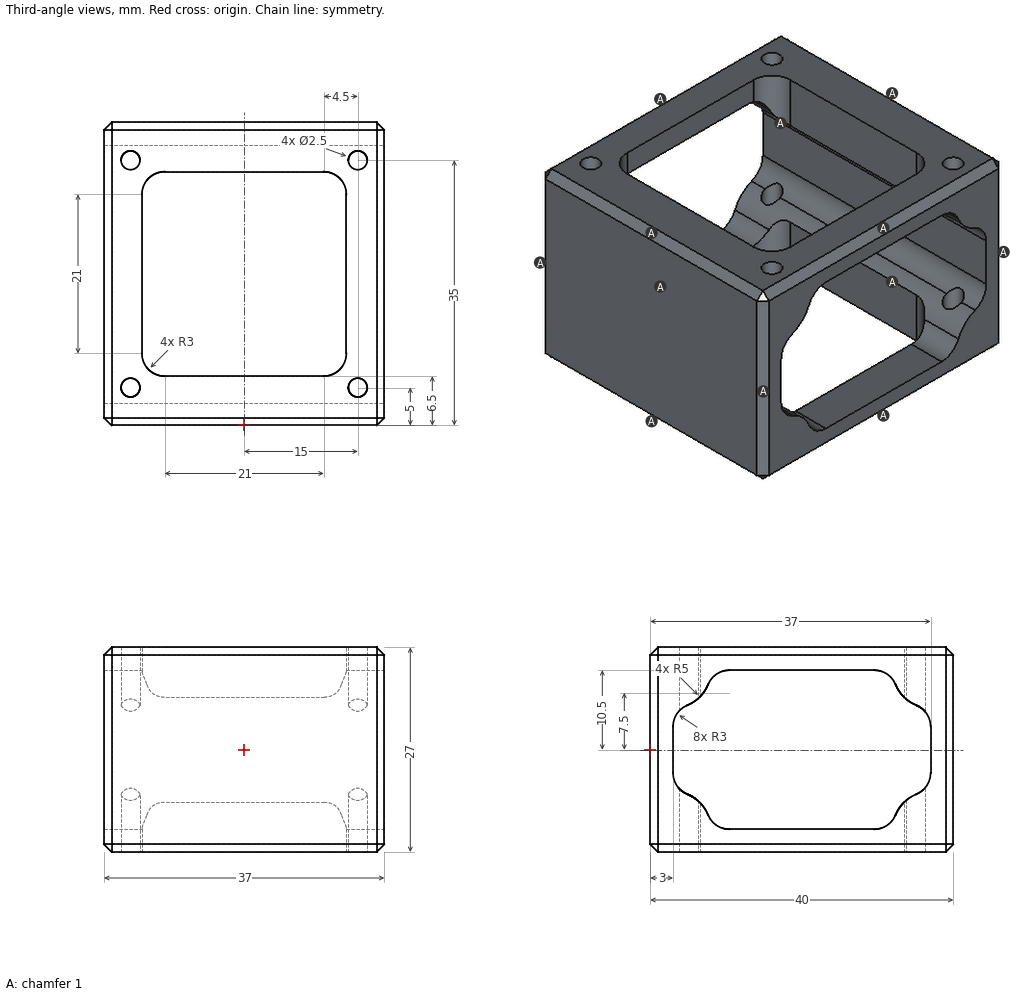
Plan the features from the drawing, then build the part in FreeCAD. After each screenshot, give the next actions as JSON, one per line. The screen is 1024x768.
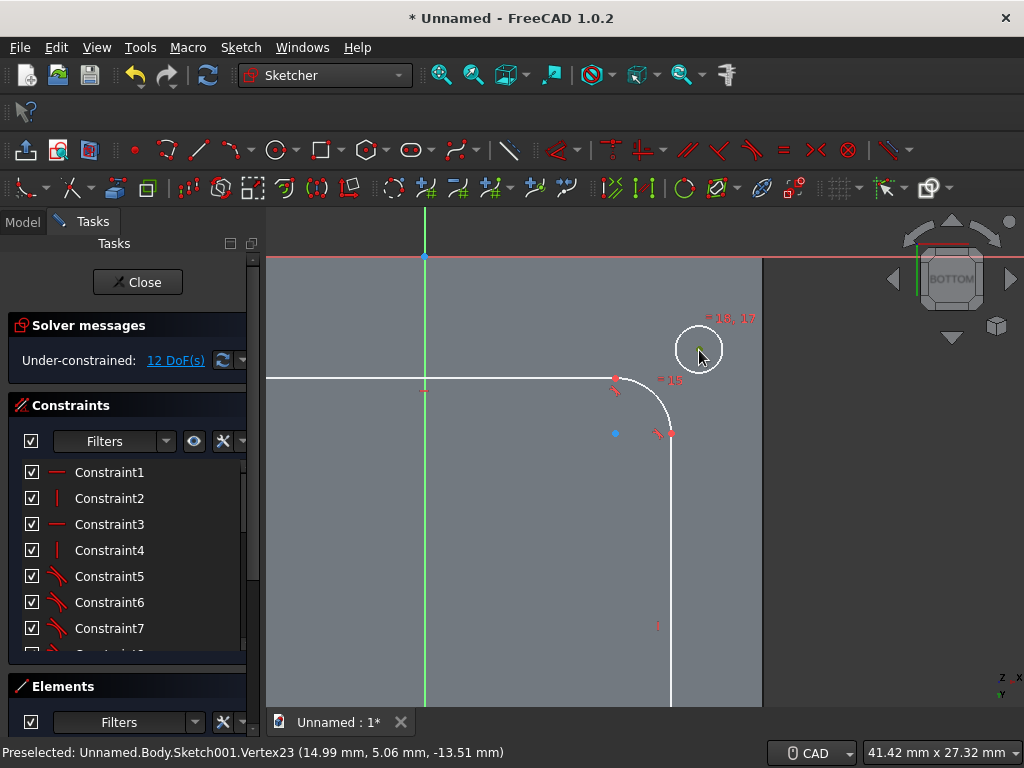
{"action": "scroll", "coordinate": [700, 350], "scroll_direction": "down", "scroll_amount": 4}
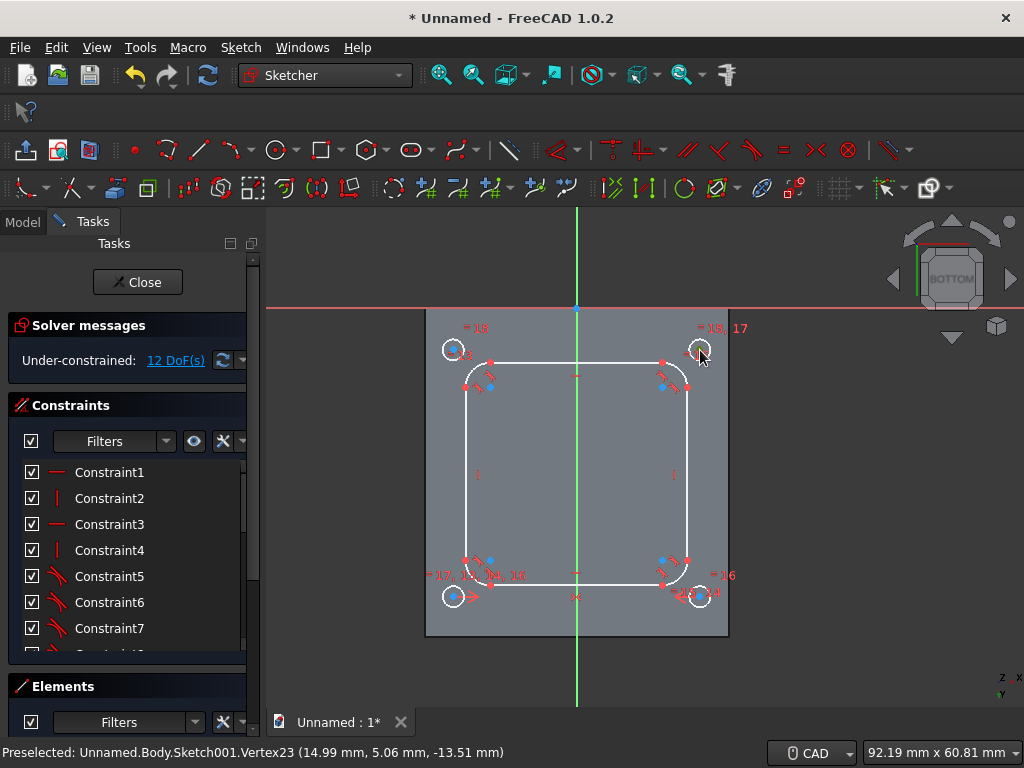
{"action": "left_click", "coordinate": [453, 350]}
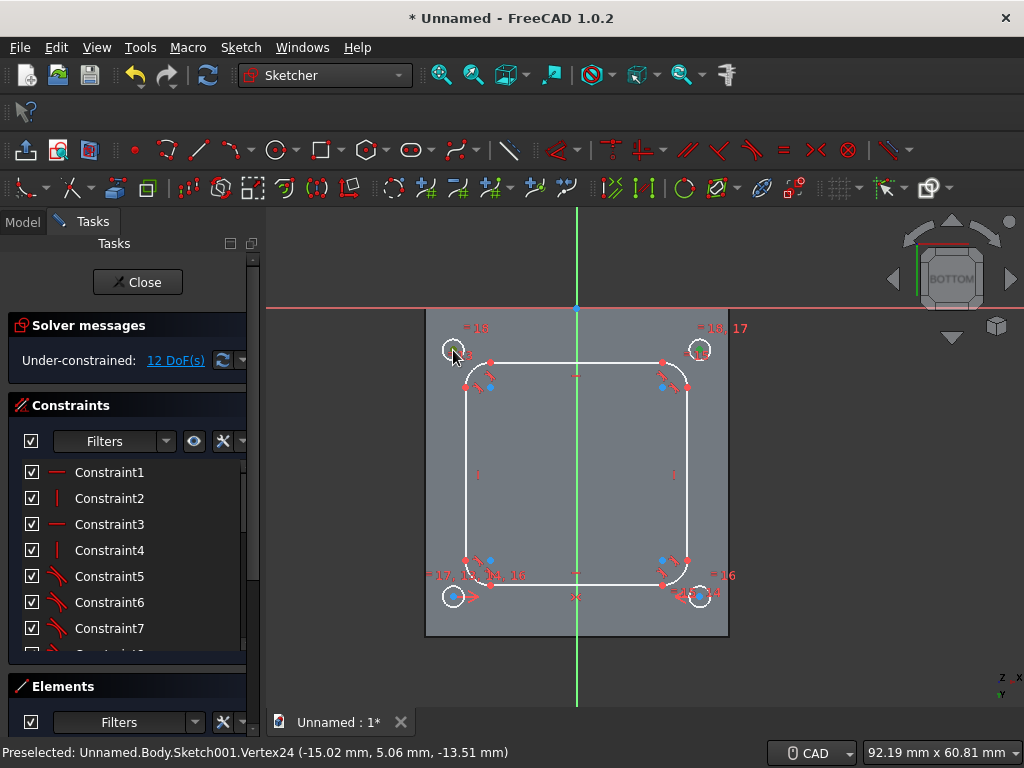
{"action": "left_click", "coordinate": [577, 647]}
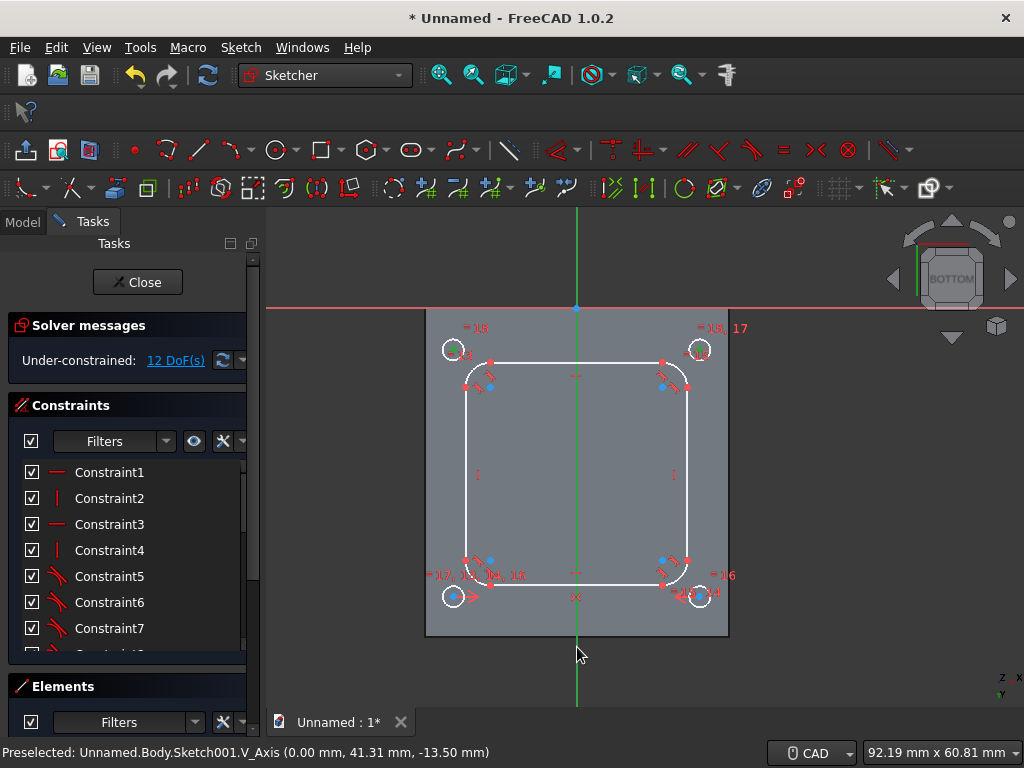
{"action": "key", "text": "s"}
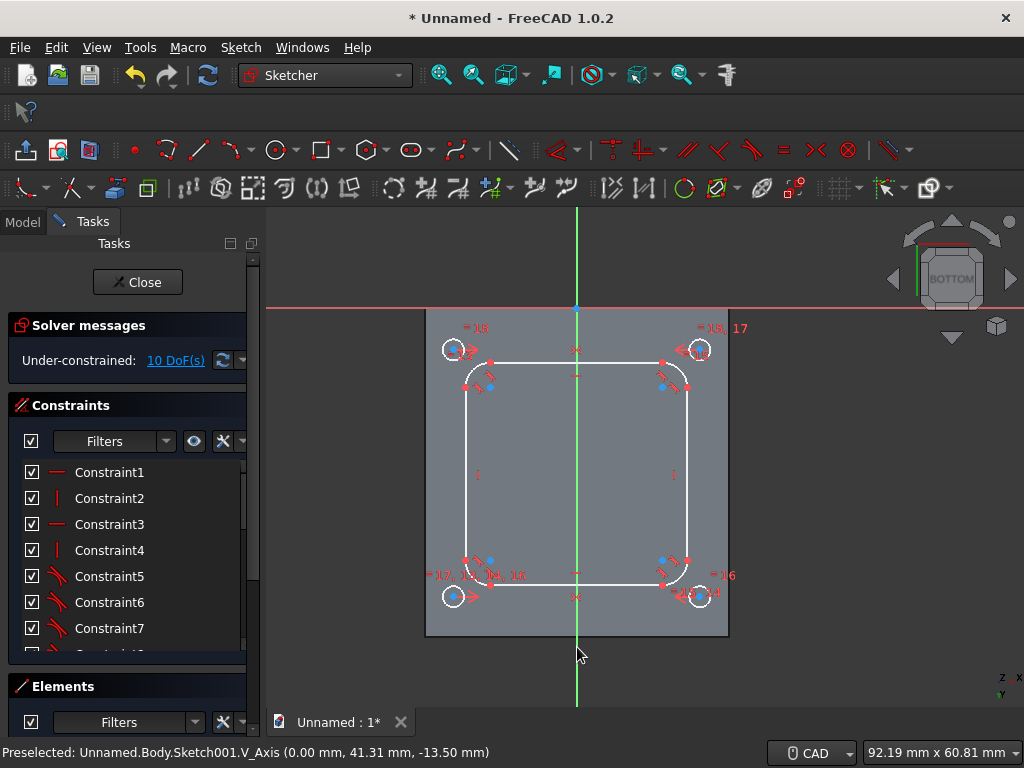
{"action": "key", "text": "d"}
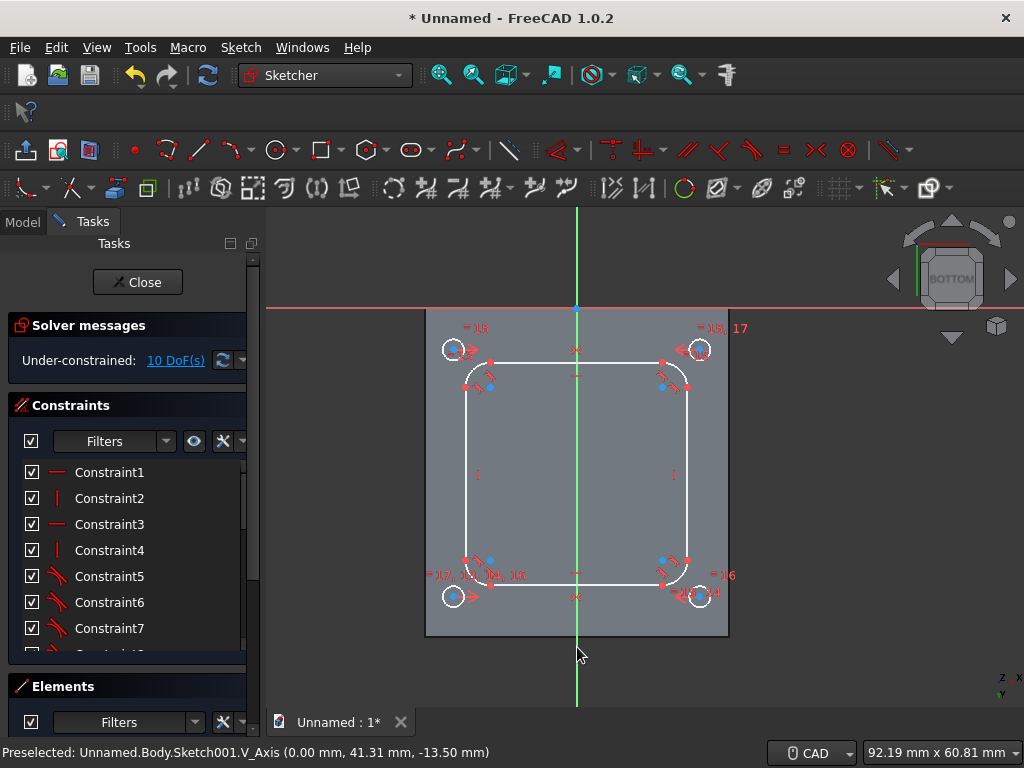
{"action": "scroll", "coordinate": [479, 365], "scroll_direction": "up", "scroll_amount": 3}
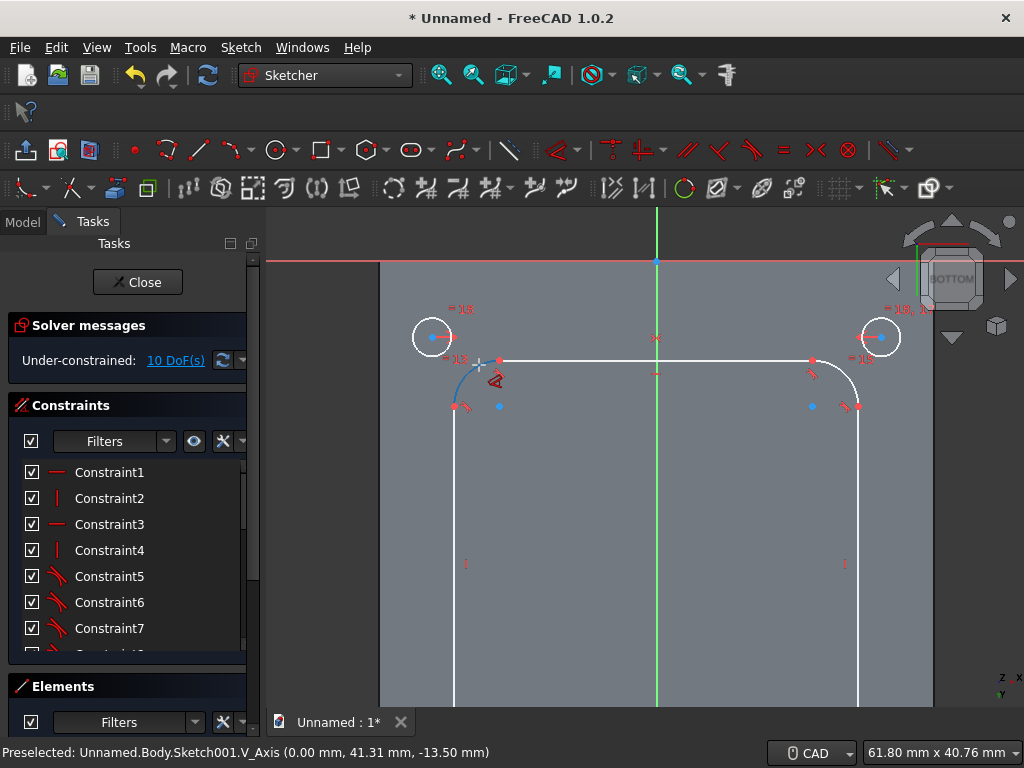
{"action": "left_click", "coordinate": [479, 366]}
{"action": "left_click", "coordinate": [464, 338]}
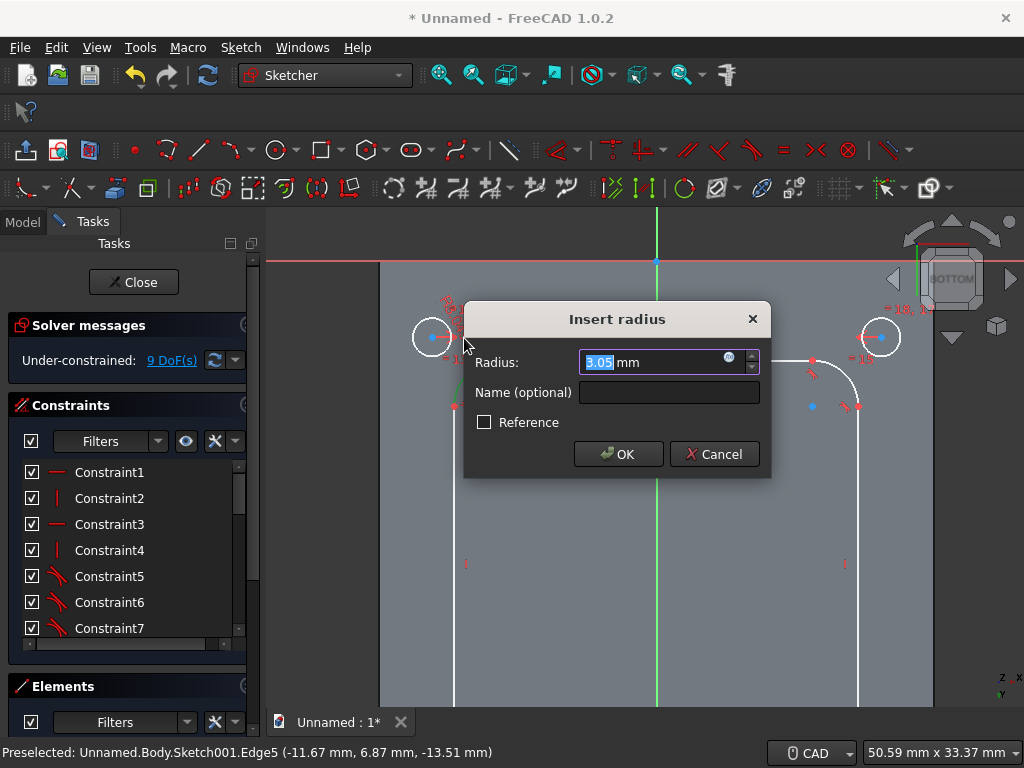
{"action": "type", "text": "3"}
{"action": "key", "text": "Return"}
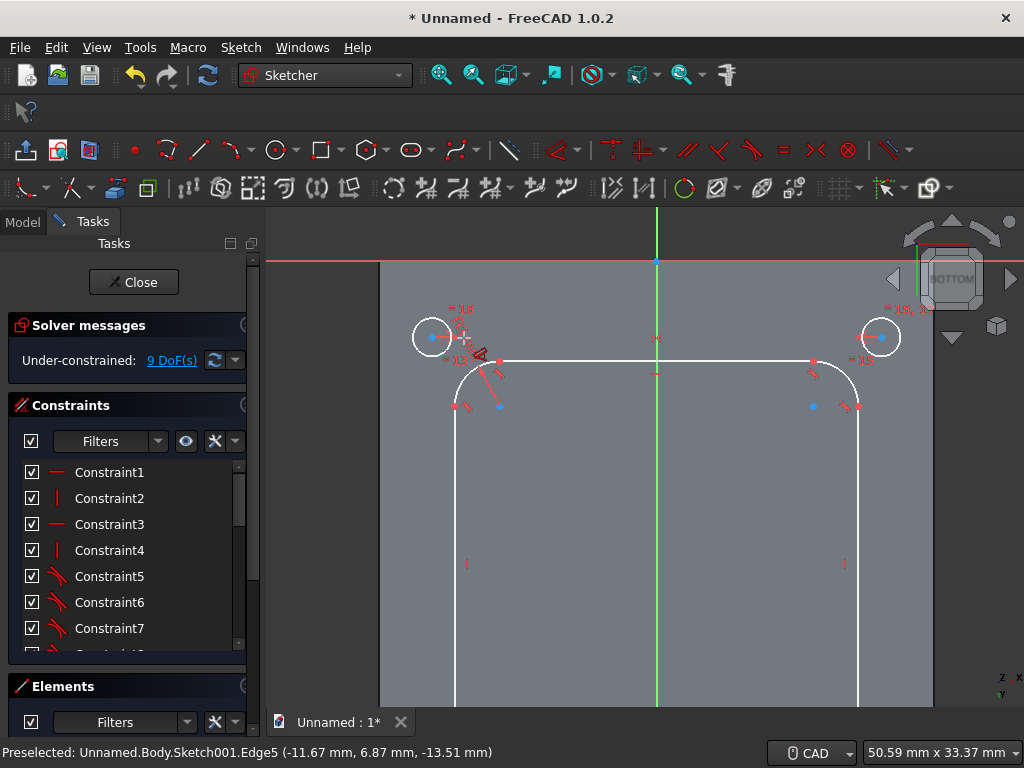
{"action": "scroll", "coordinate": [479, 365], "scroll_direction": "down", "scroll_amount": 3}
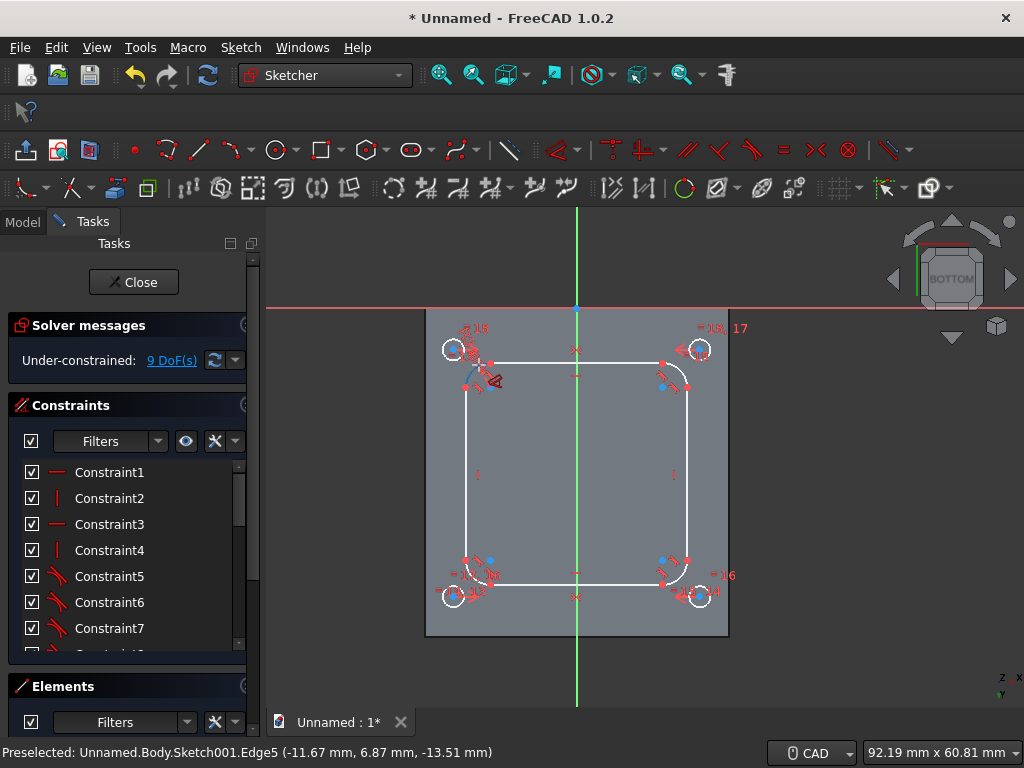
{"action": "scroll", "coordinate": [707, 589], "scroll_direction": "up", "scroll_amount": 4}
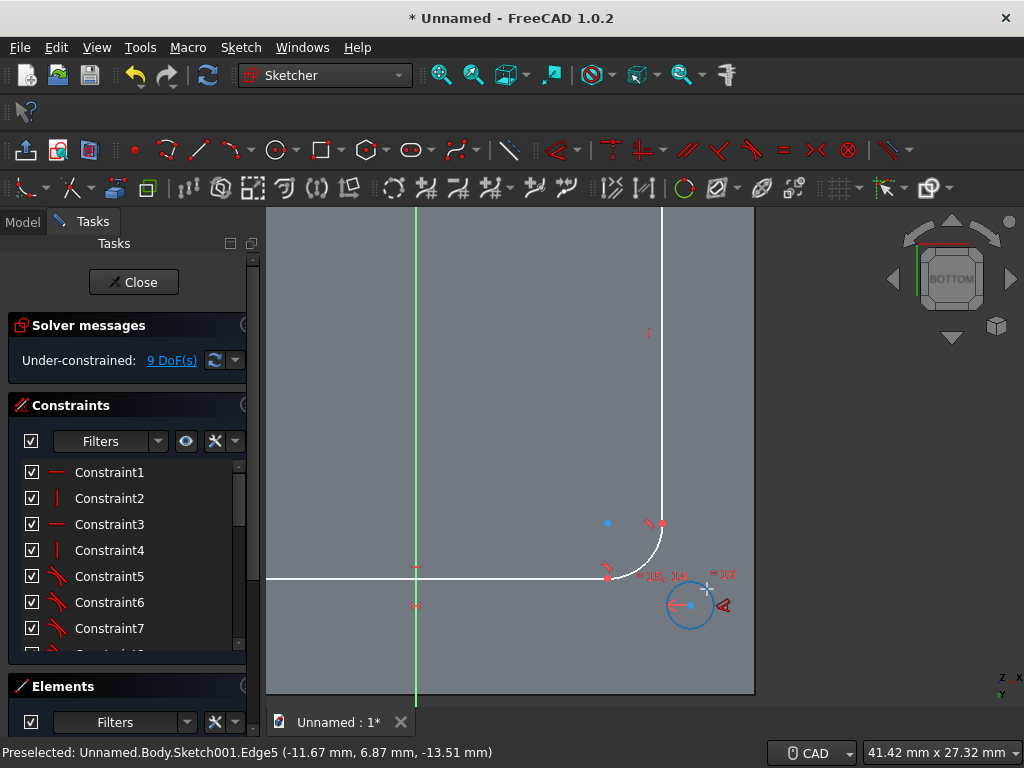
{"action": "left_click", "coordinate": [707, 589]}
{"action": "left_click", "coordinate": [730, 567]}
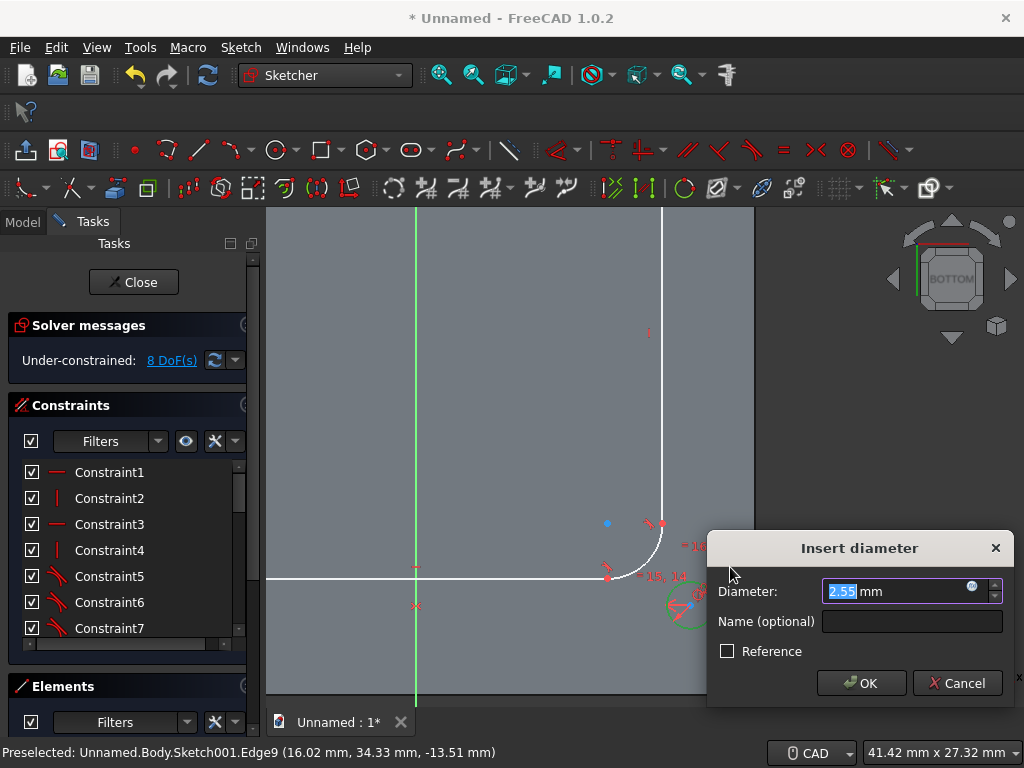
{"action": "type", "text": "2.5"}
{"action": "key", "text": "Return"}